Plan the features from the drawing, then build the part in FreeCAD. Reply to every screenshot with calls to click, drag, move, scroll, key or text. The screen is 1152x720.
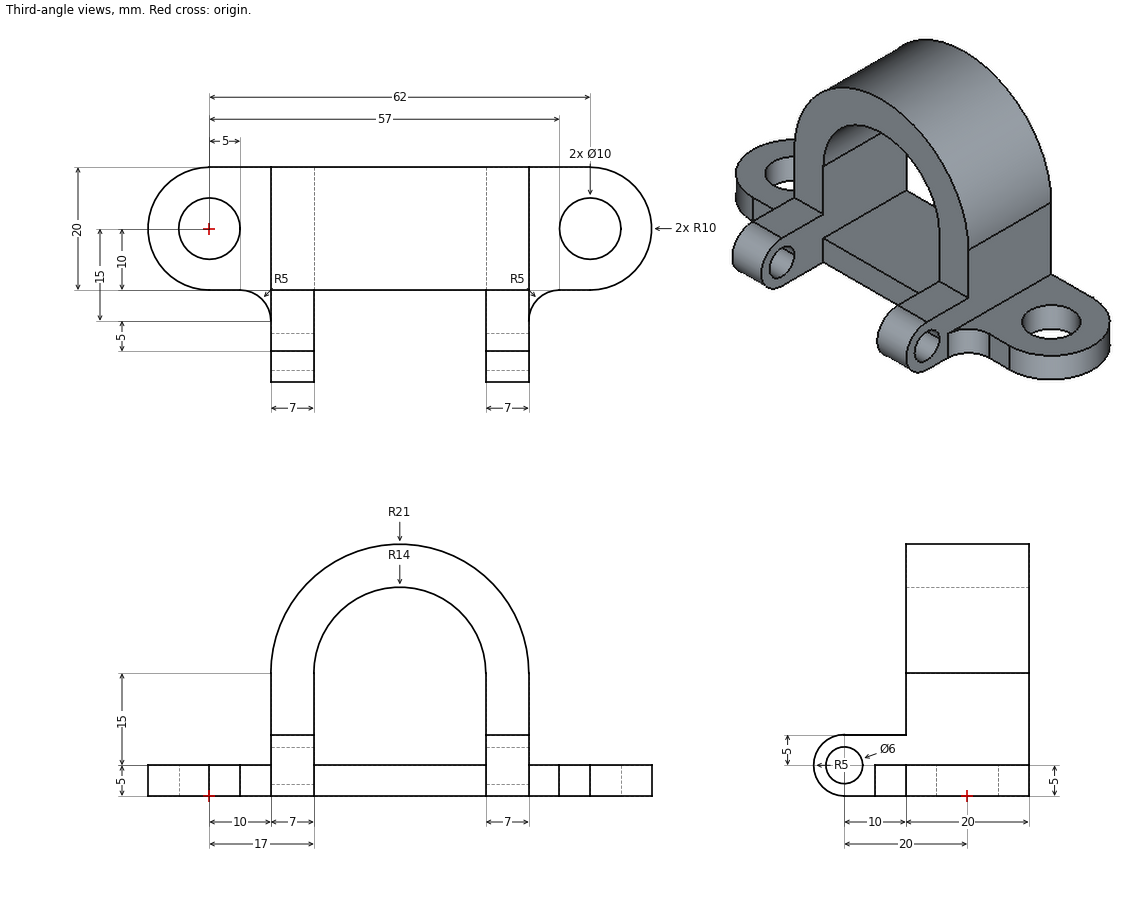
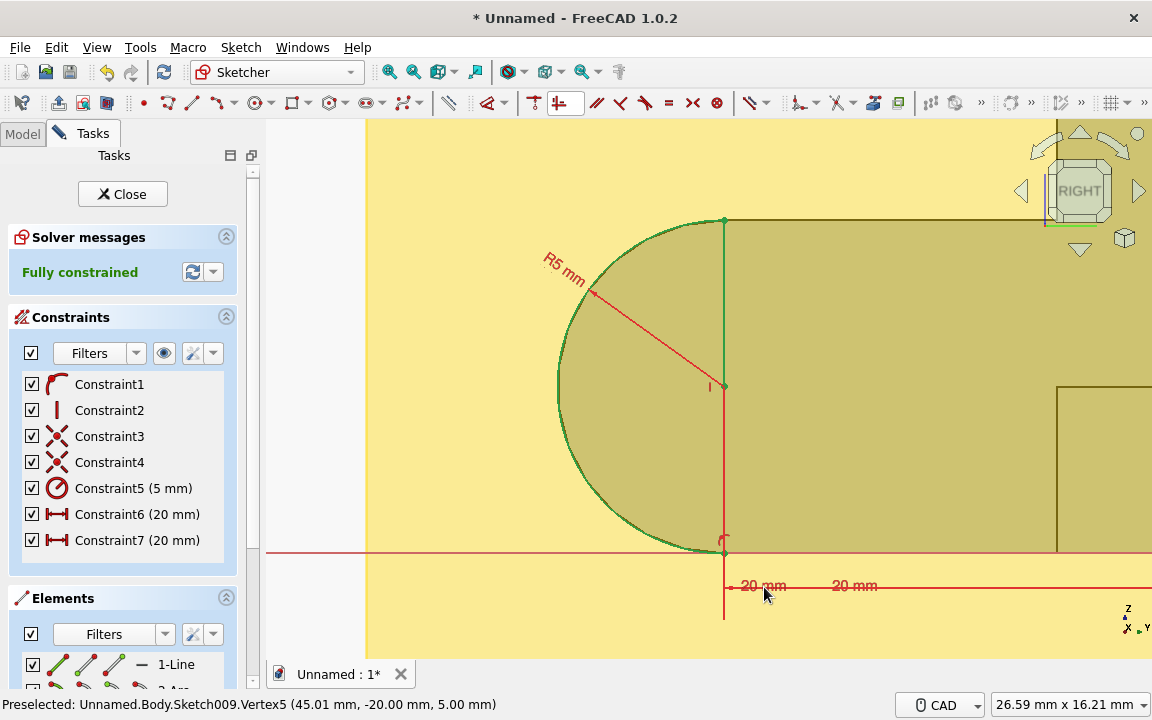
click(123, 194)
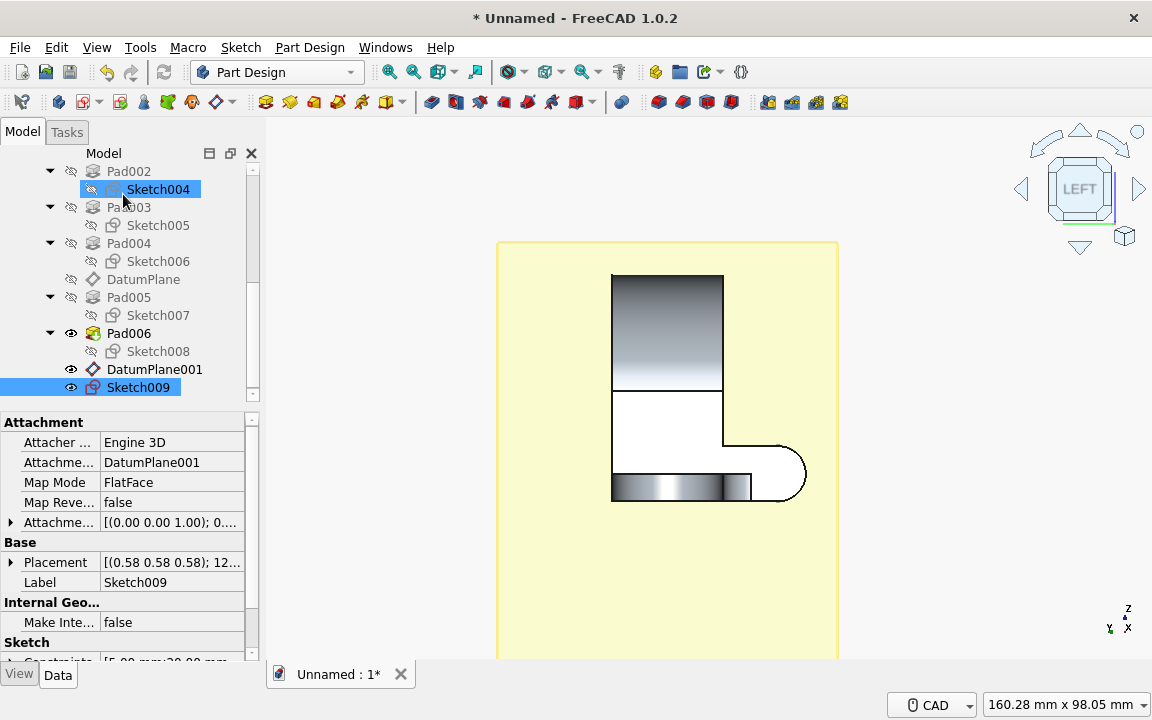
click(266, 102)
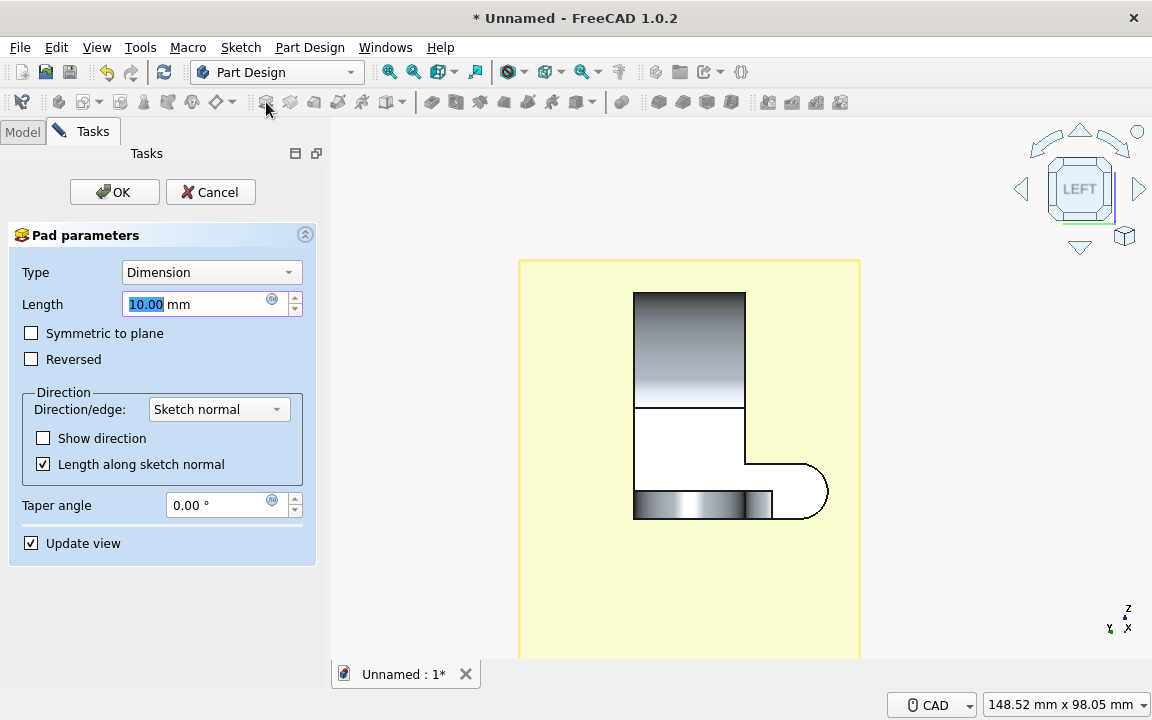
text(7)
key(Tab)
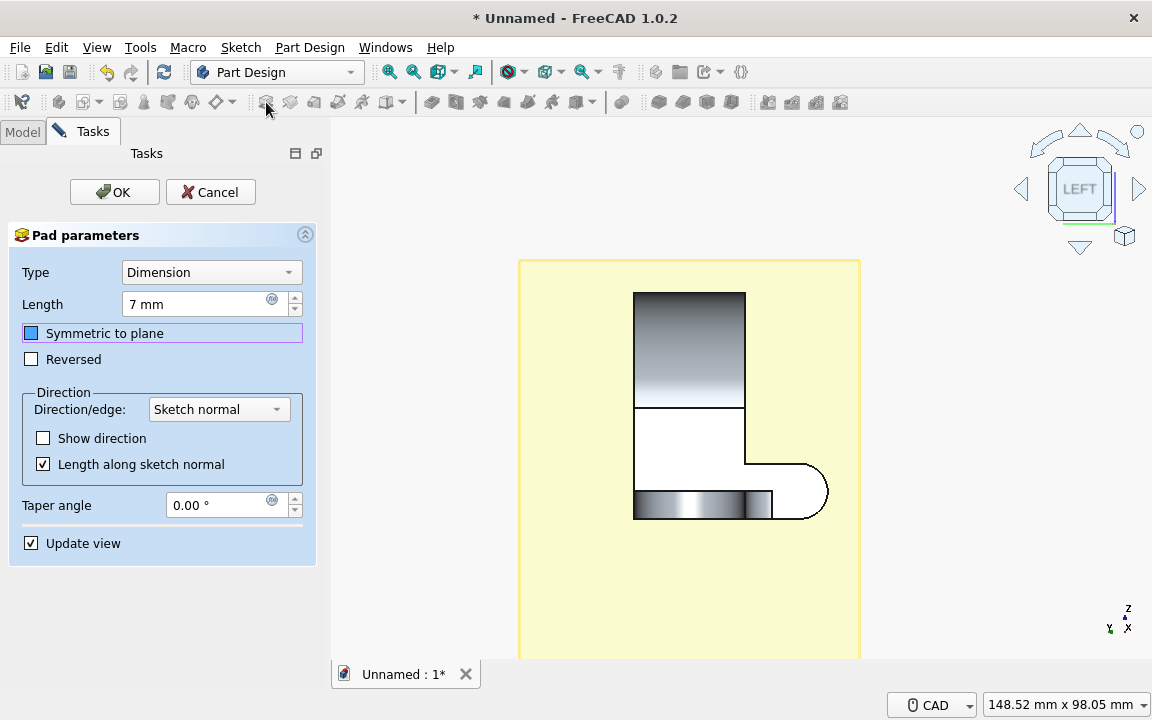
click(115, 192)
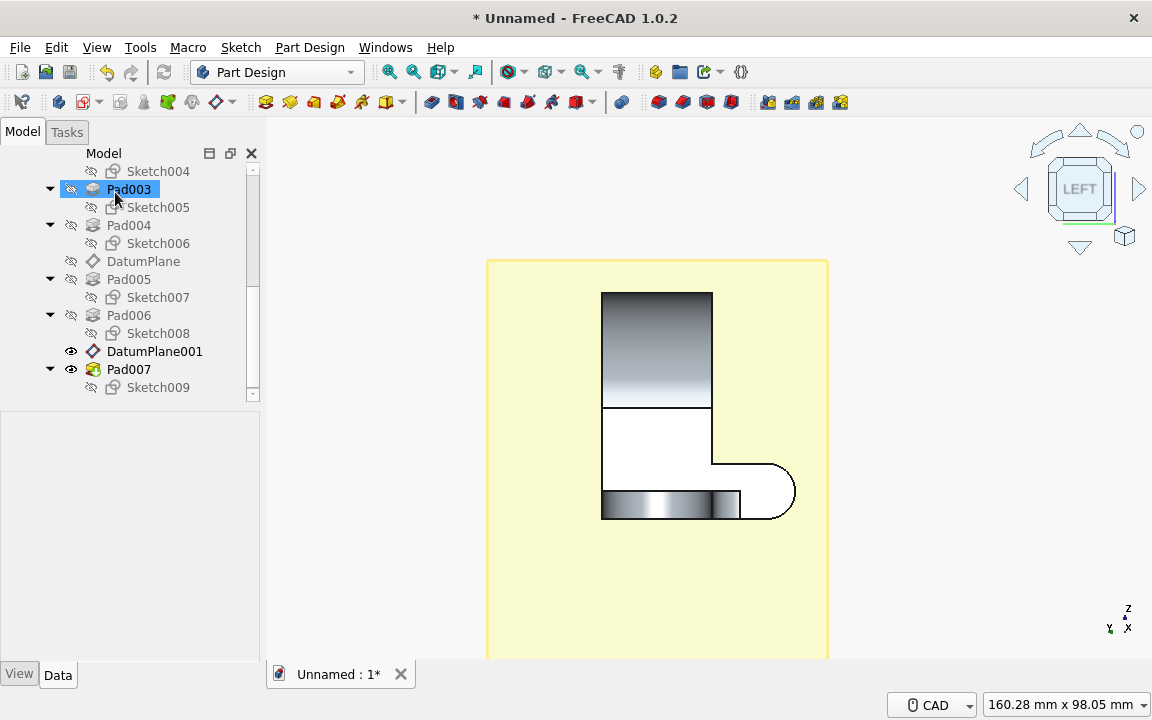
click(116, 351)
key(space)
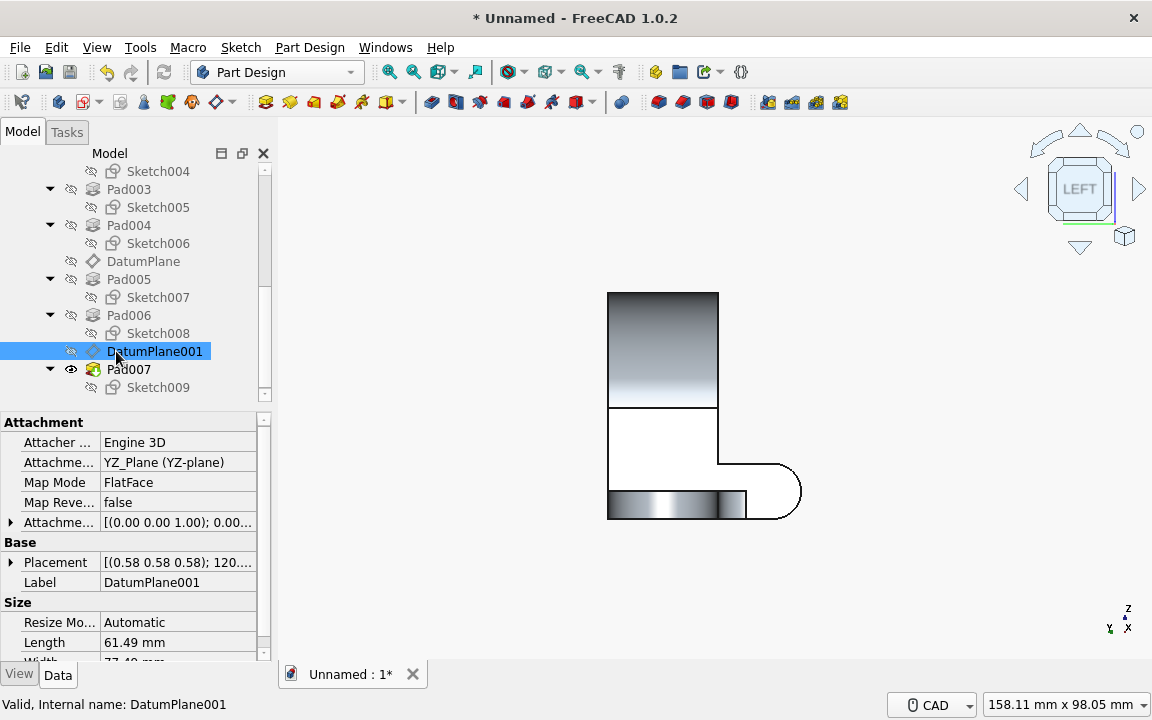
key(v)
key(f)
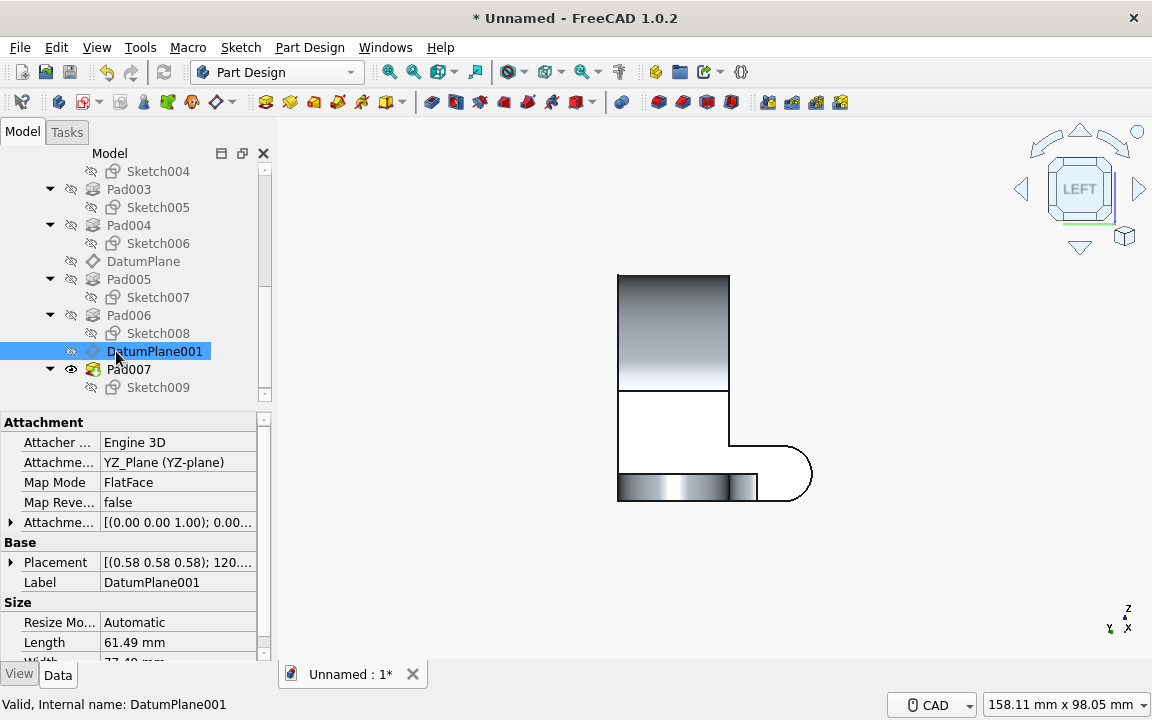
key(0)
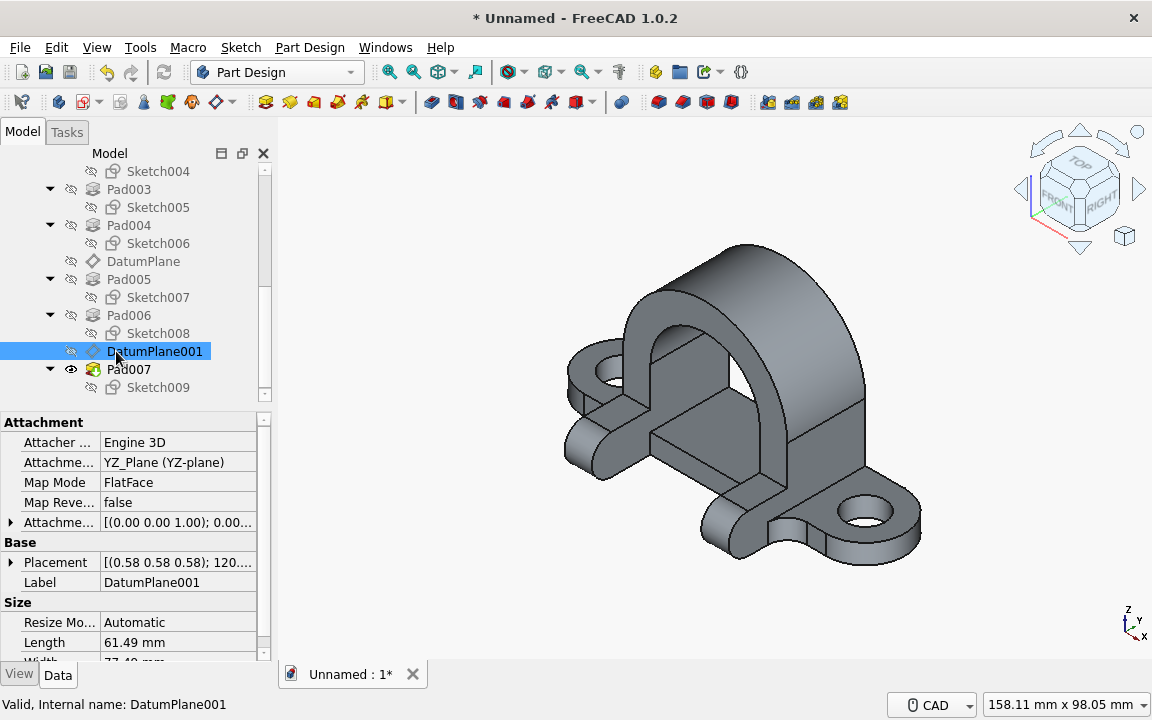
click(817, 458)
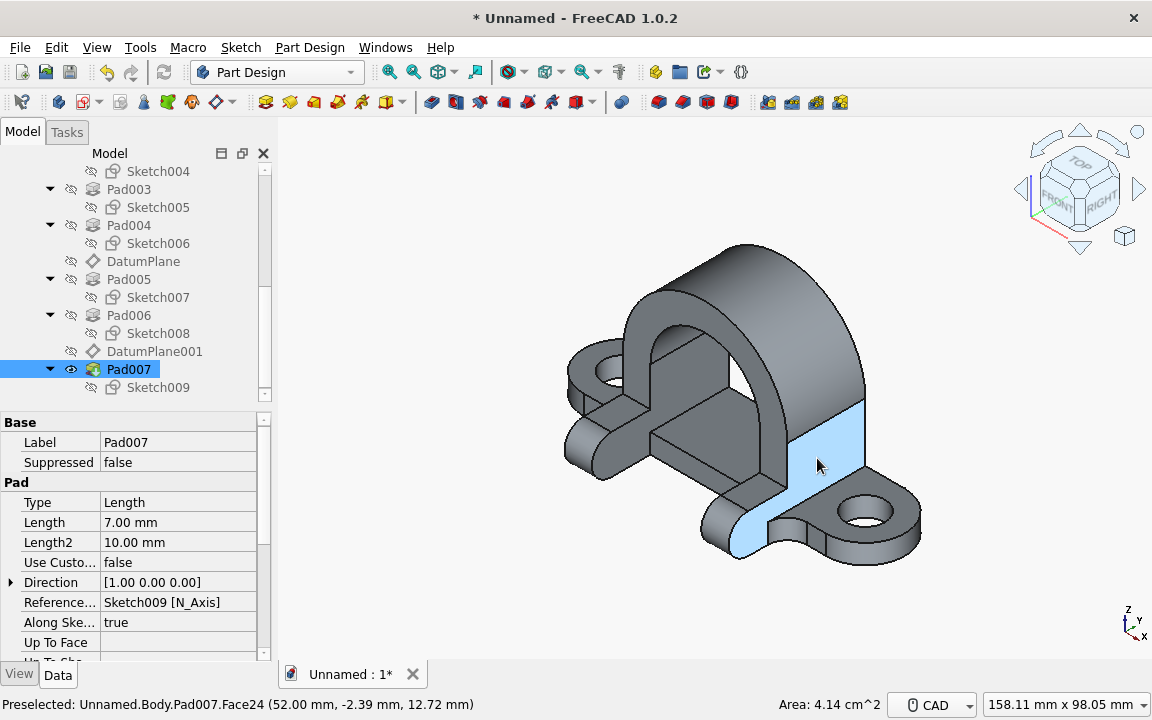
click(84, 102)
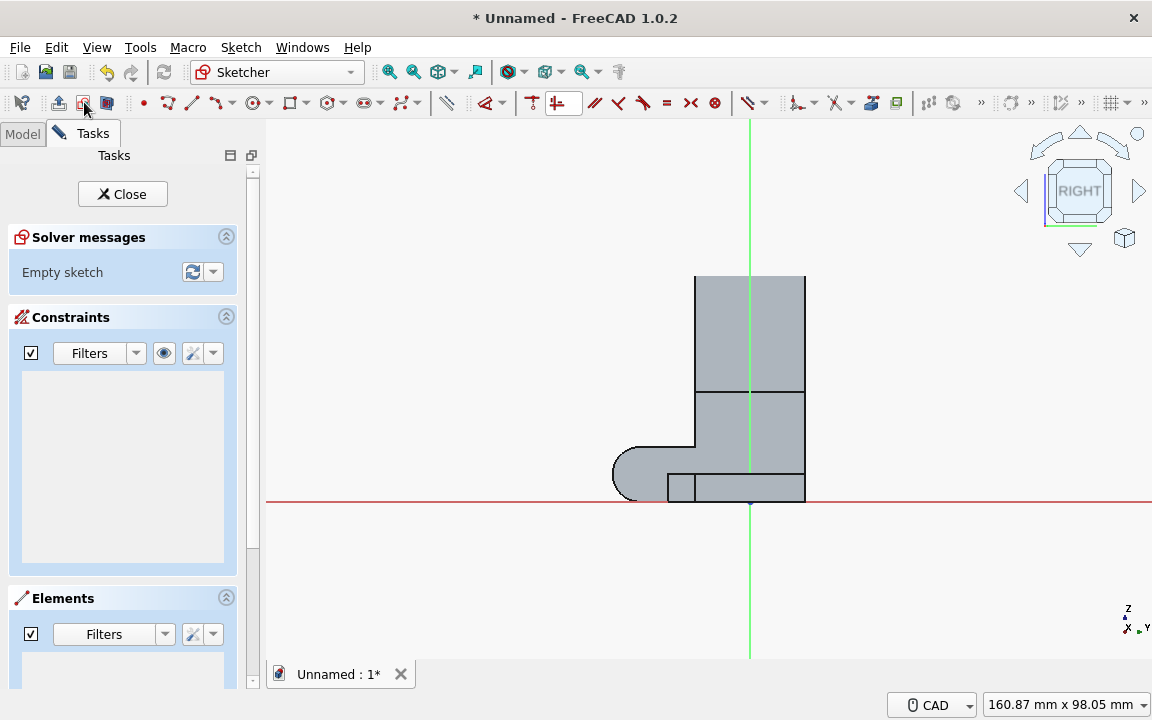
scroll(640, 483, up, 12)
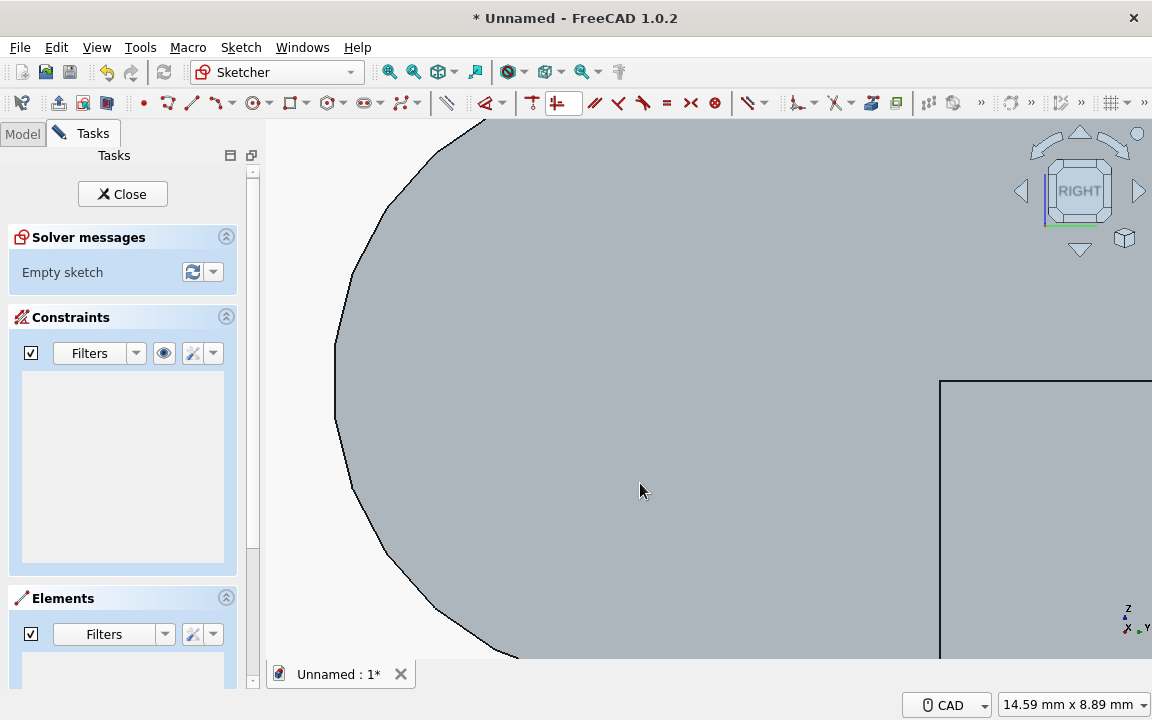
click(254, 104)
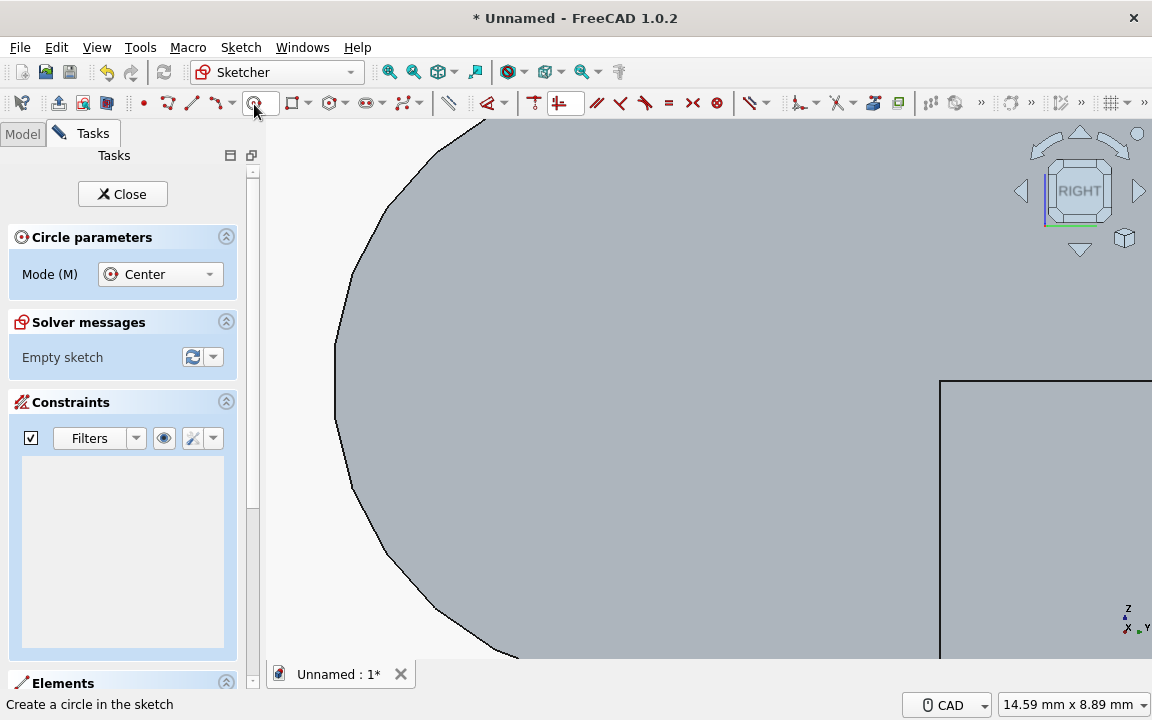
click(636, 381)
move(765, 252)